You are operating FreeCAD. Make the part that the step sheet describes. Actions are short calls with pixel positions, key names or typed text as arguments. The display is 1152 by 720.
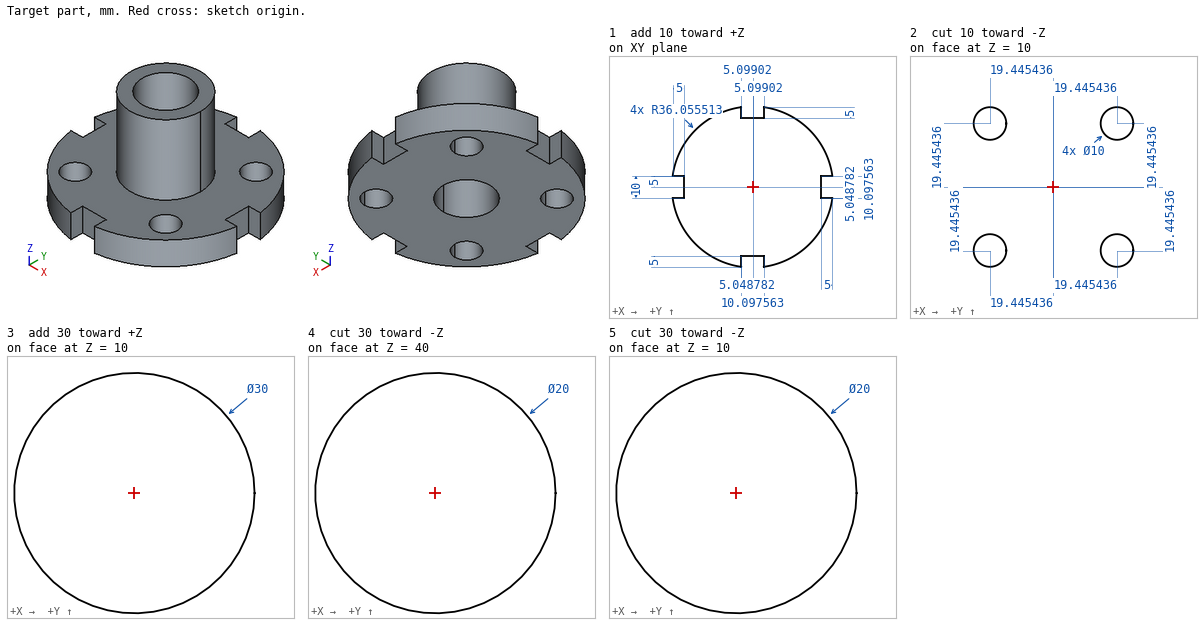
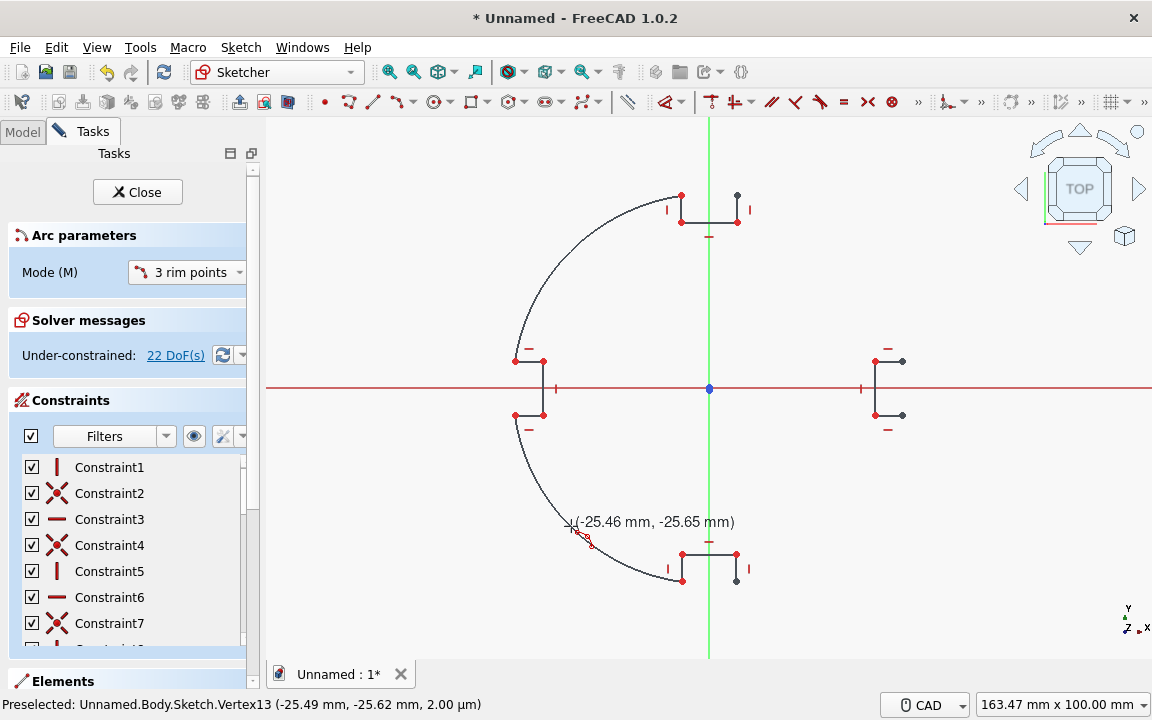
click(736, 582)
click(902, 416)
click(847, 526)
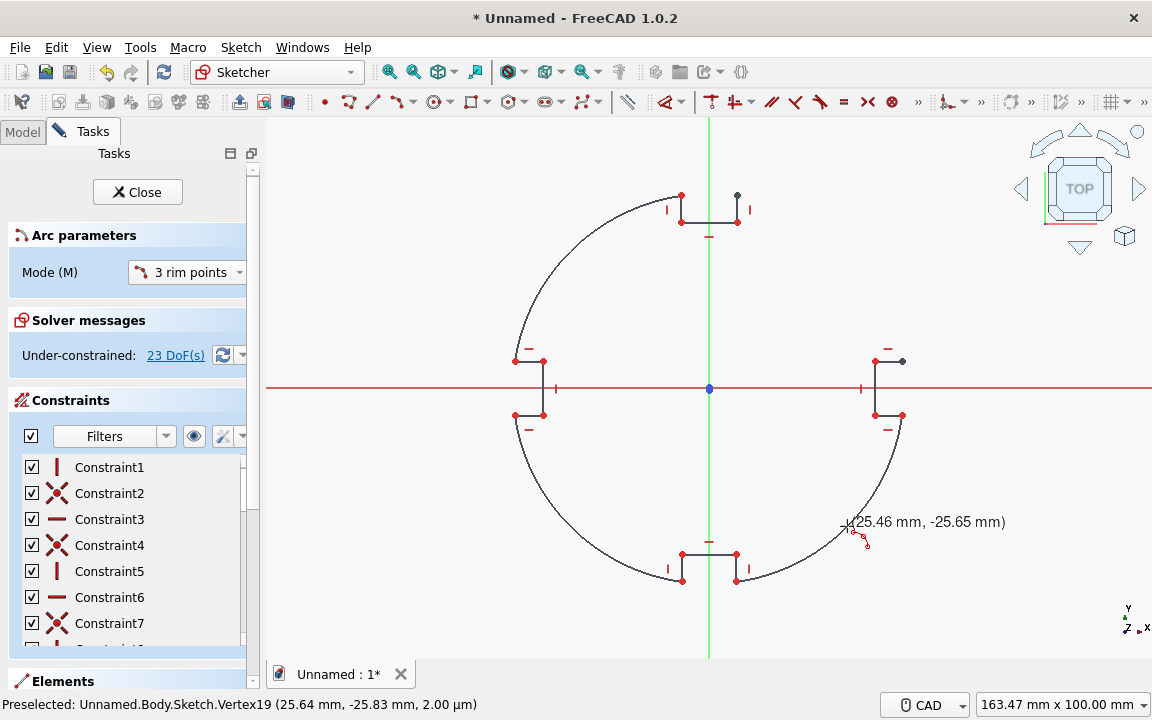
click(902, 362)
click(737, 196)
click(847, 250)
key(Escape)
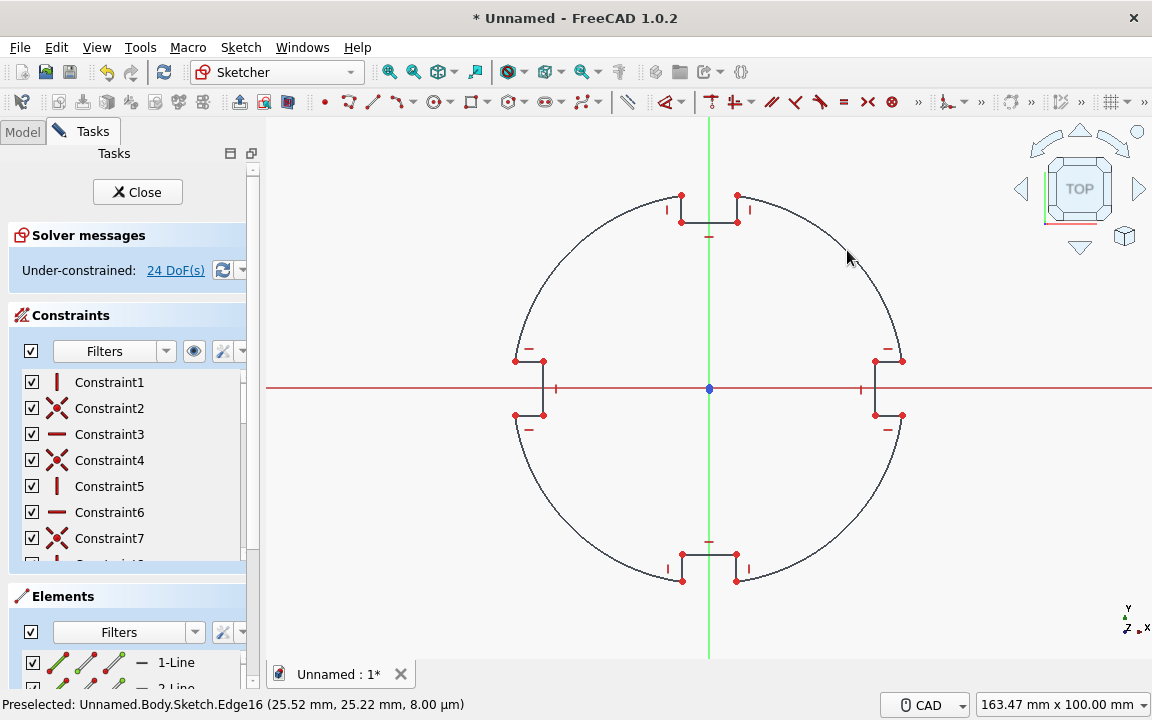
click(610, 221)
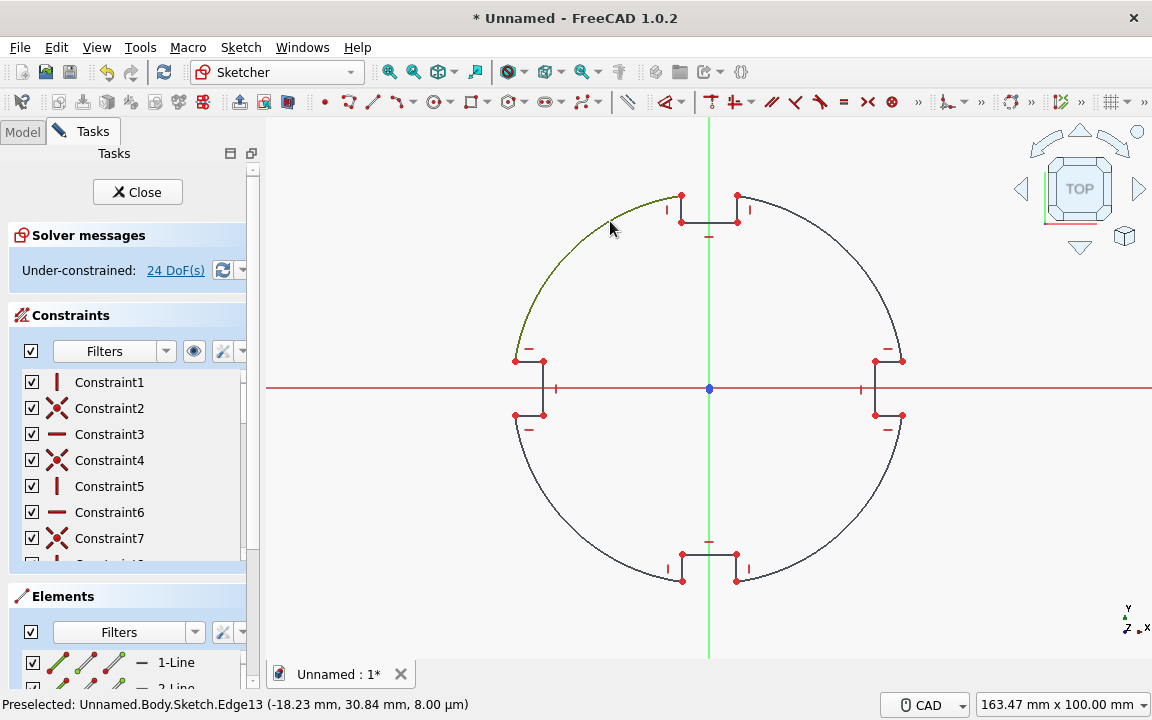
click(540, 487)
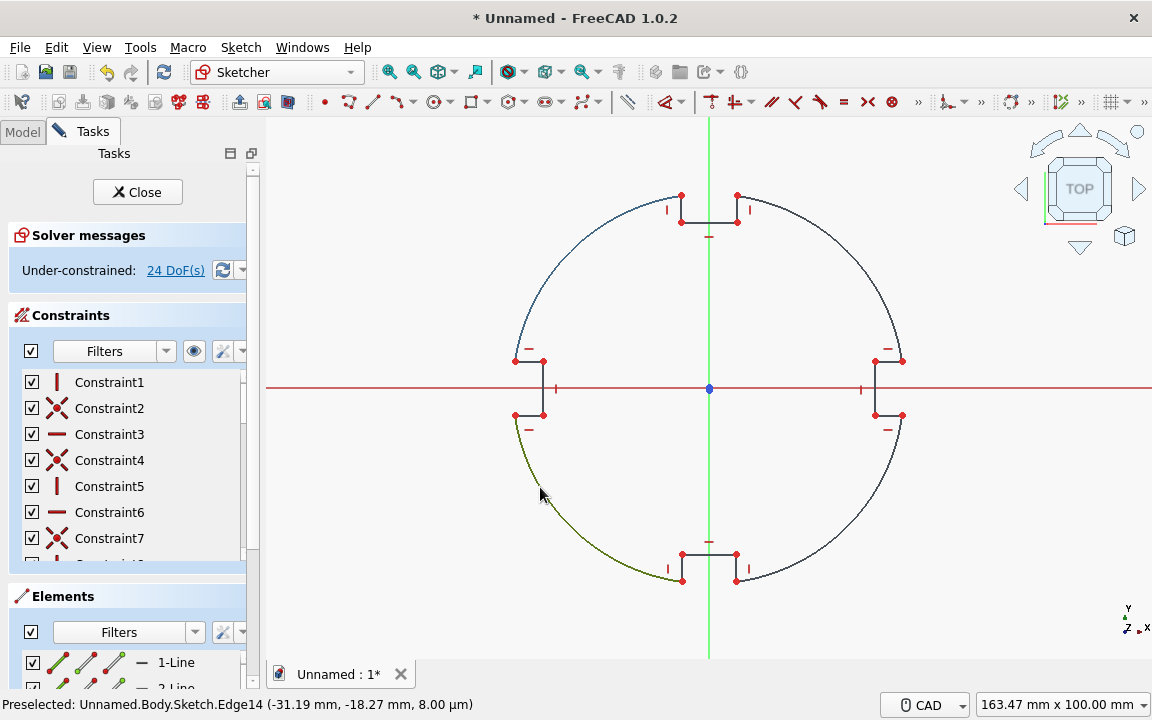
key(c)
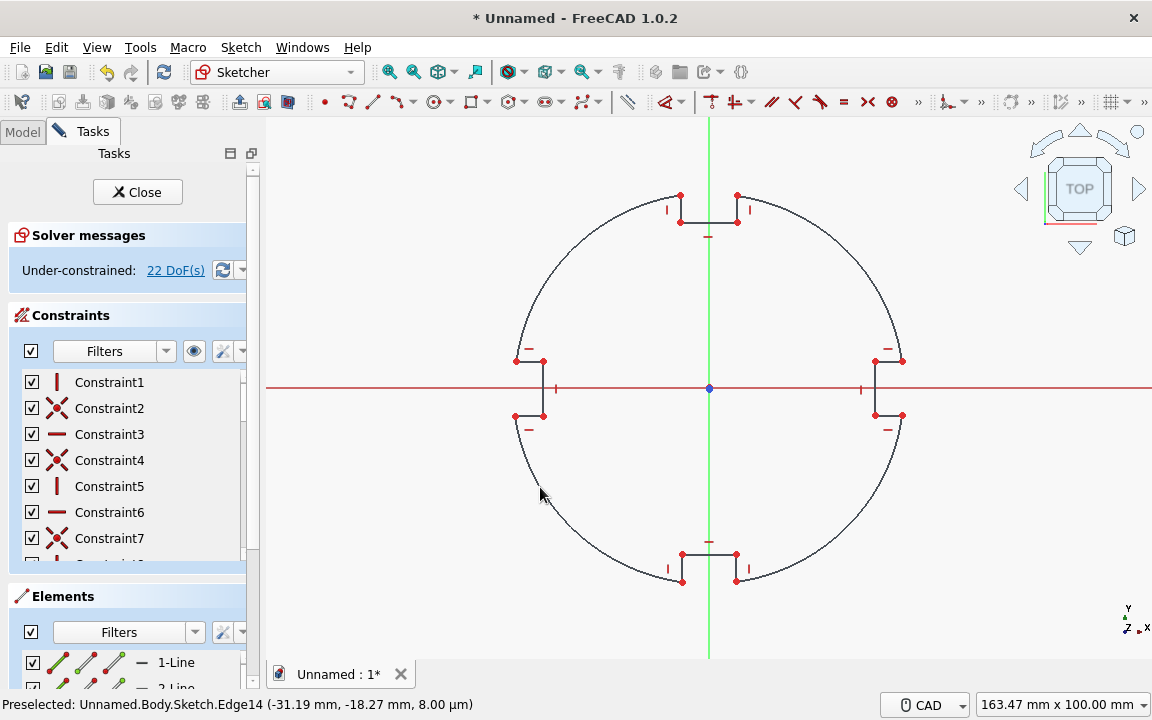
click(610, 220)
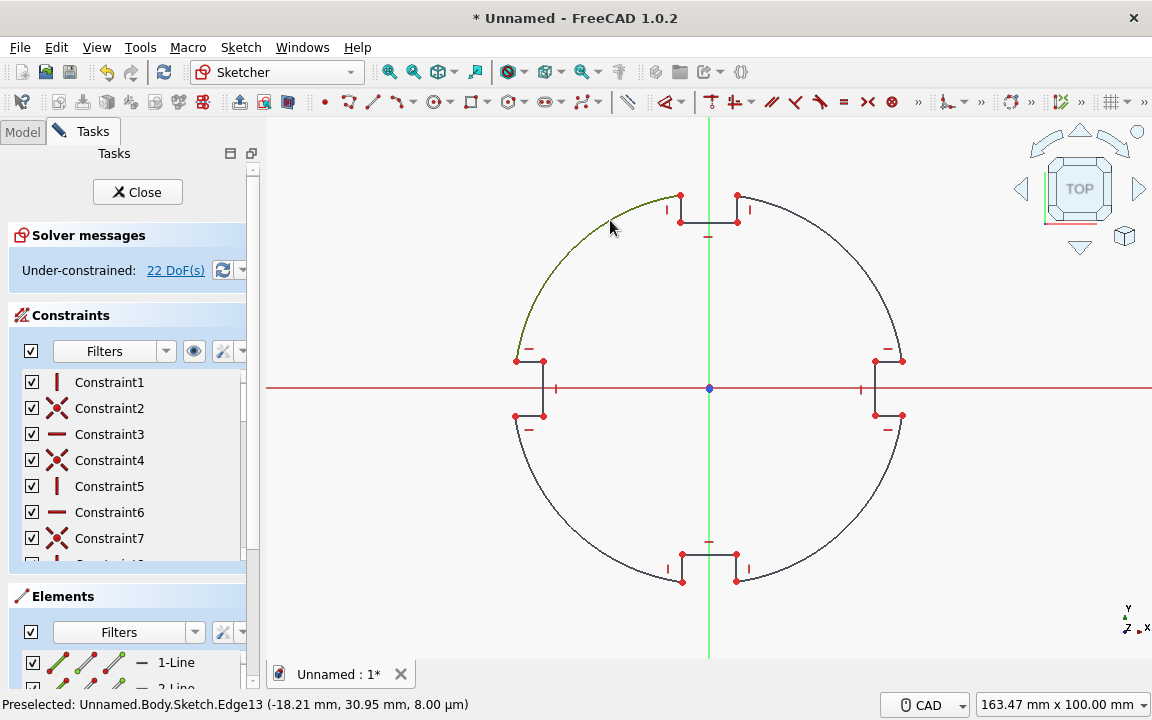
click(807, 558)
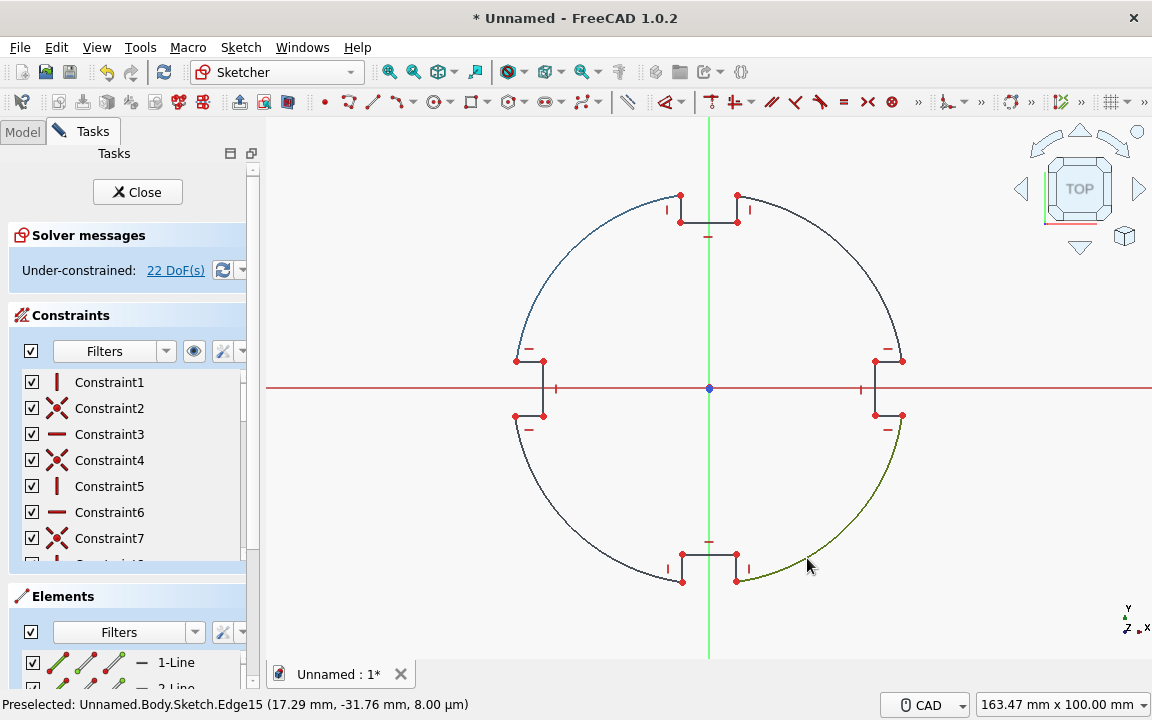
click(712, 102)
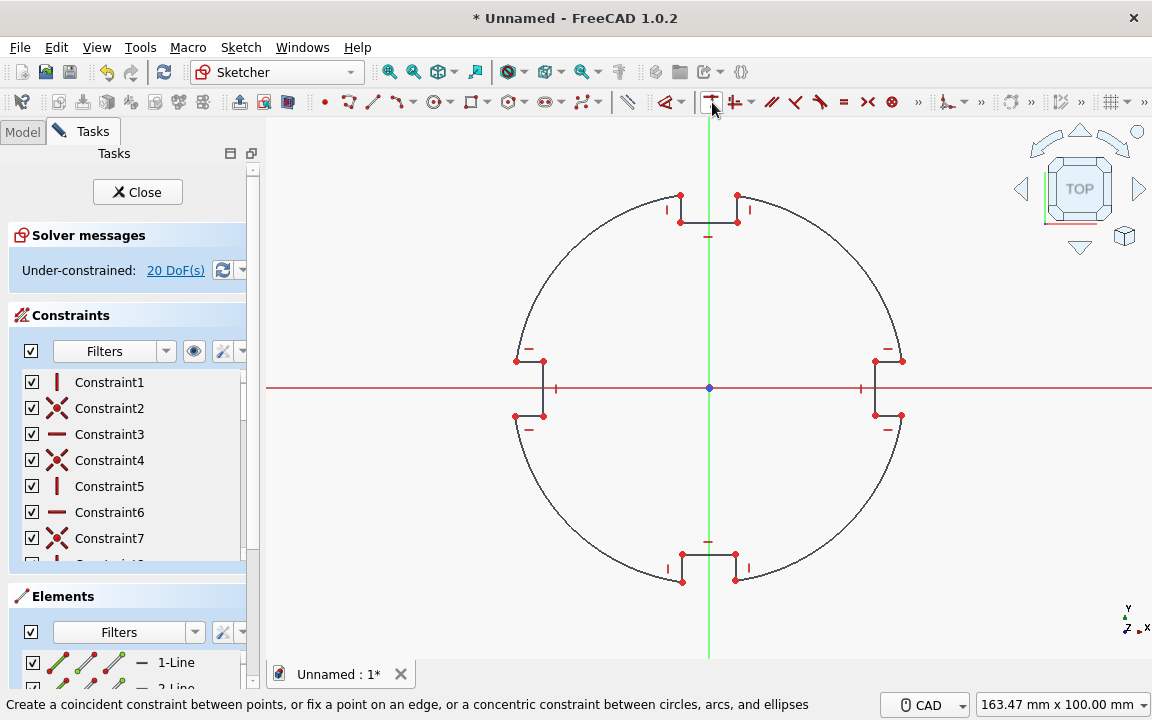
click(610, 220)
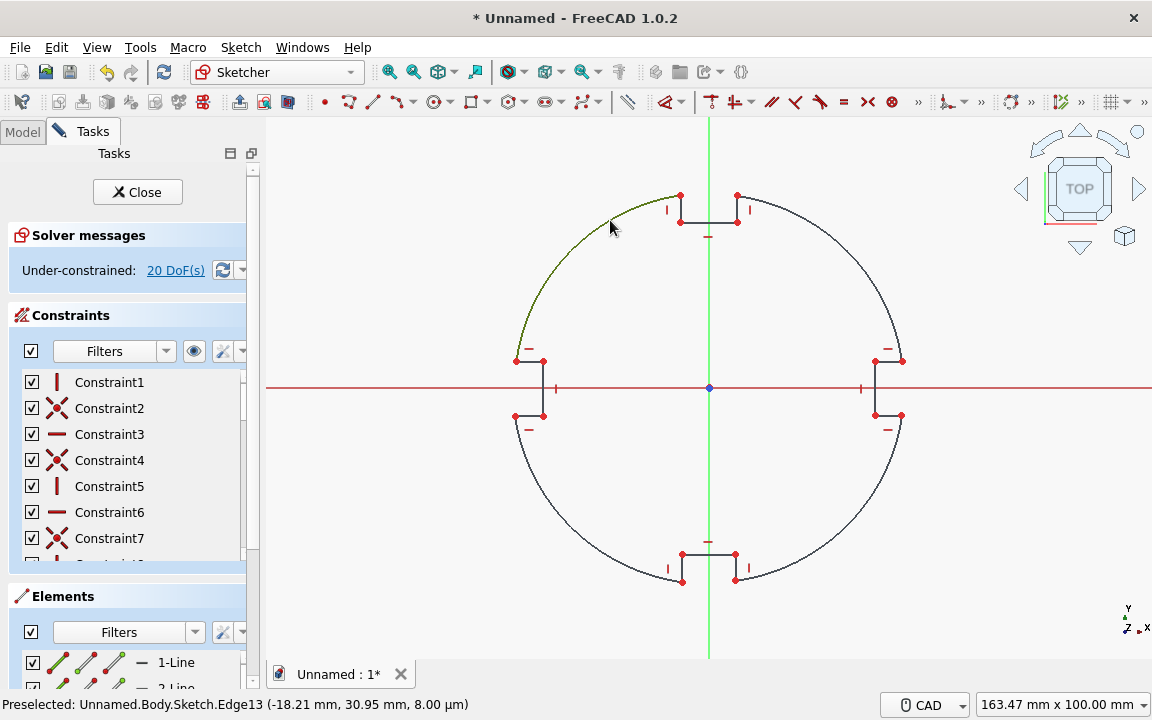
click(878, 291)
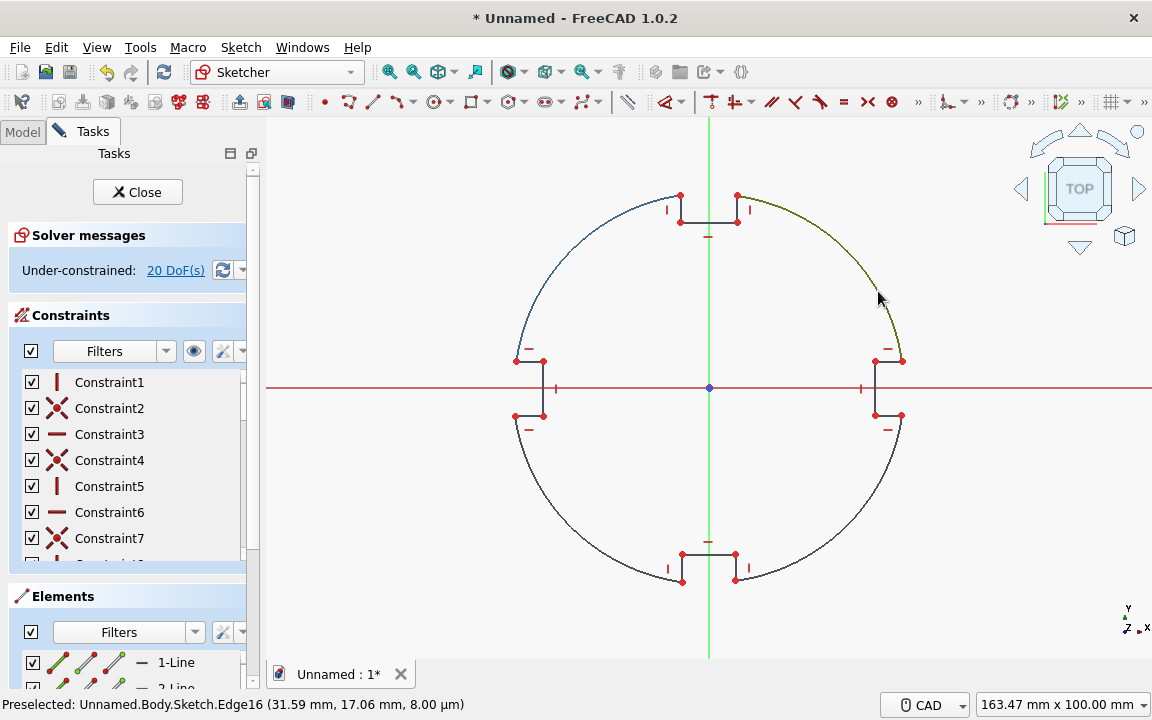
click(712, 102)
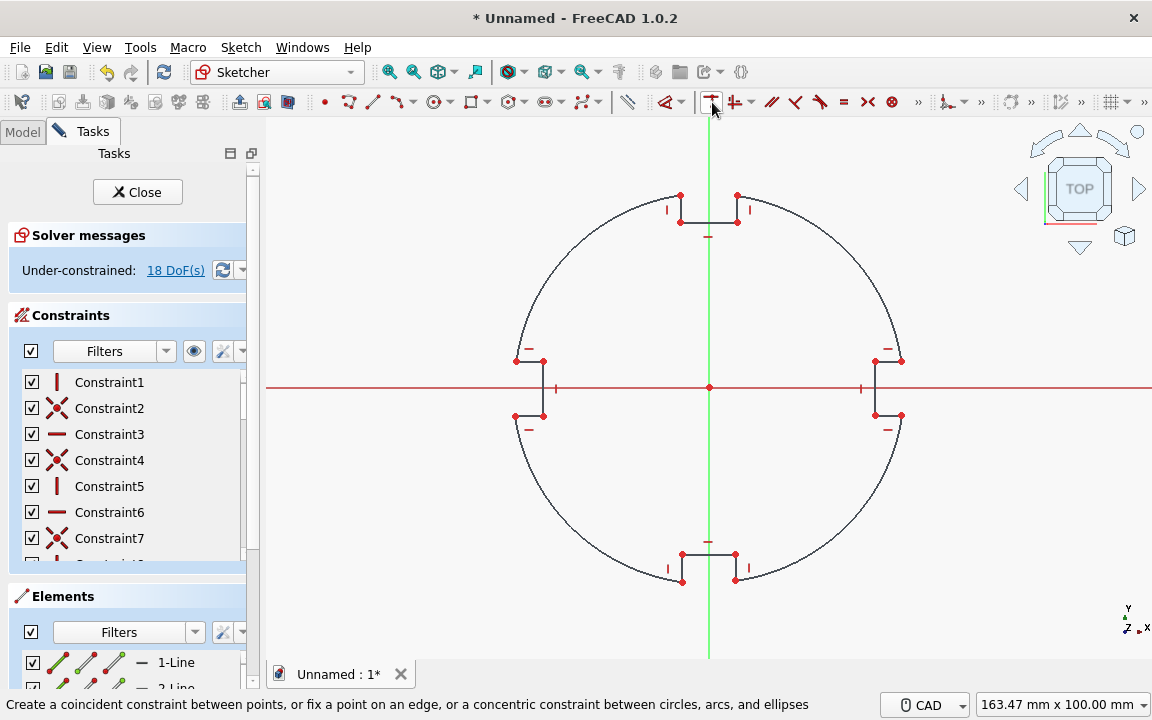
drag(699, 378, 719, 398)